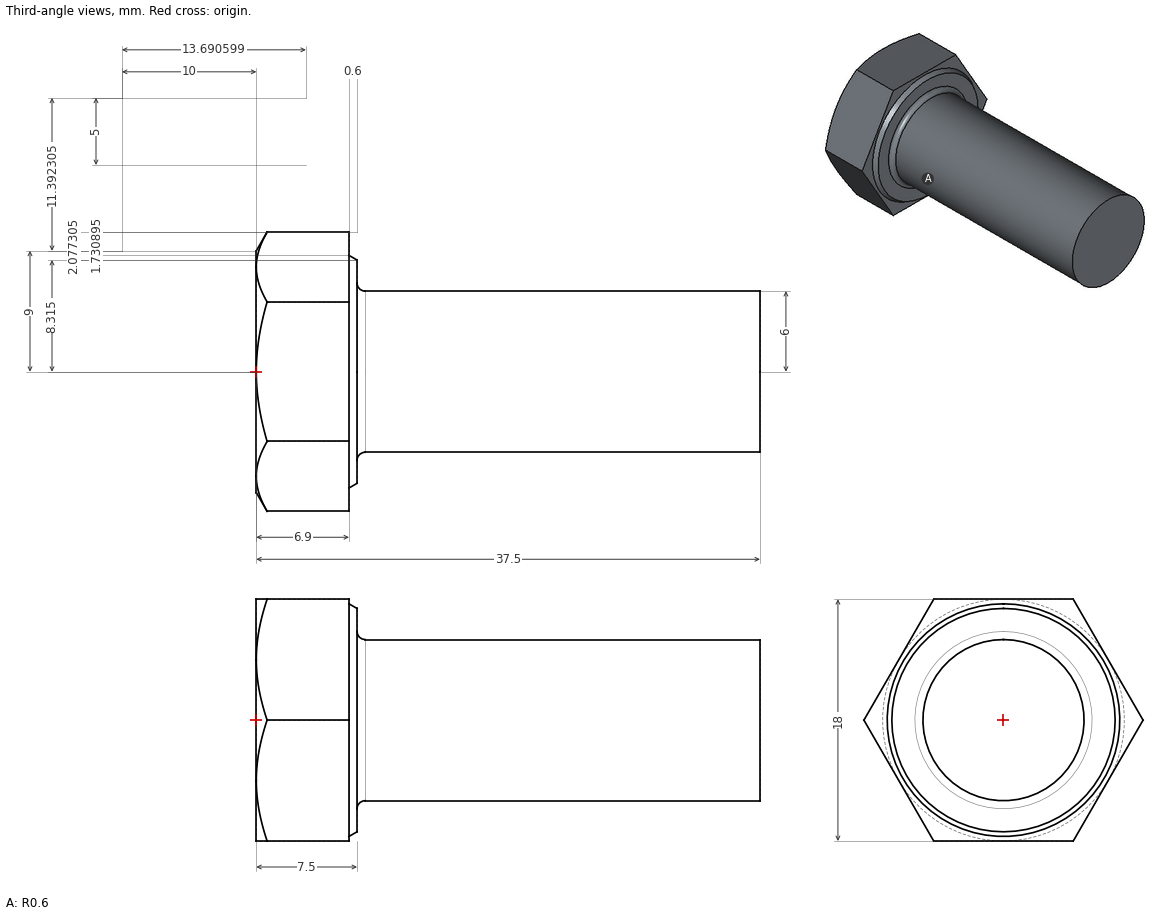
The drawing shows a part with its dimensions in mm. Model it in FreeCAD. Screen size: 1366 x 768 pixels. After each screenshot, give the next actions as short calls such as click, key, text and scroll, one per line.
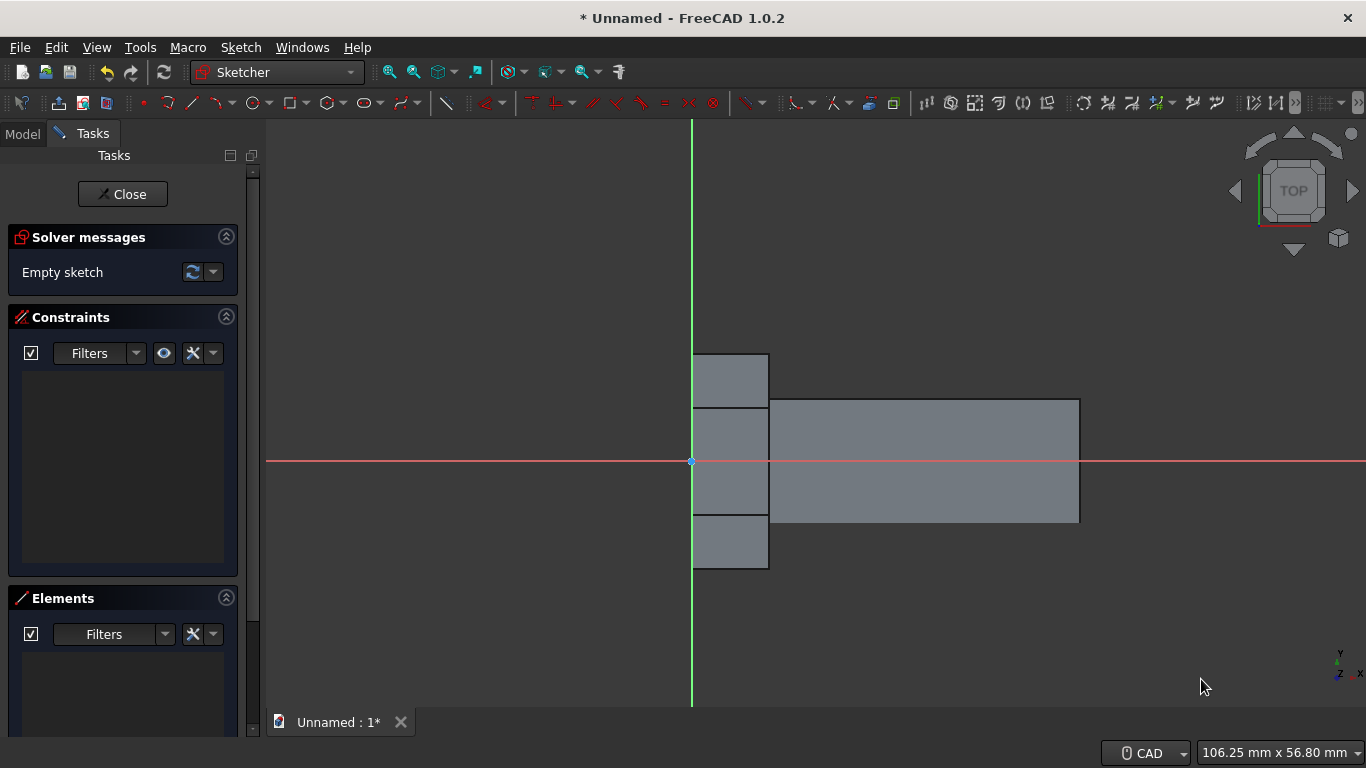
scroll(552, 286, up, 3)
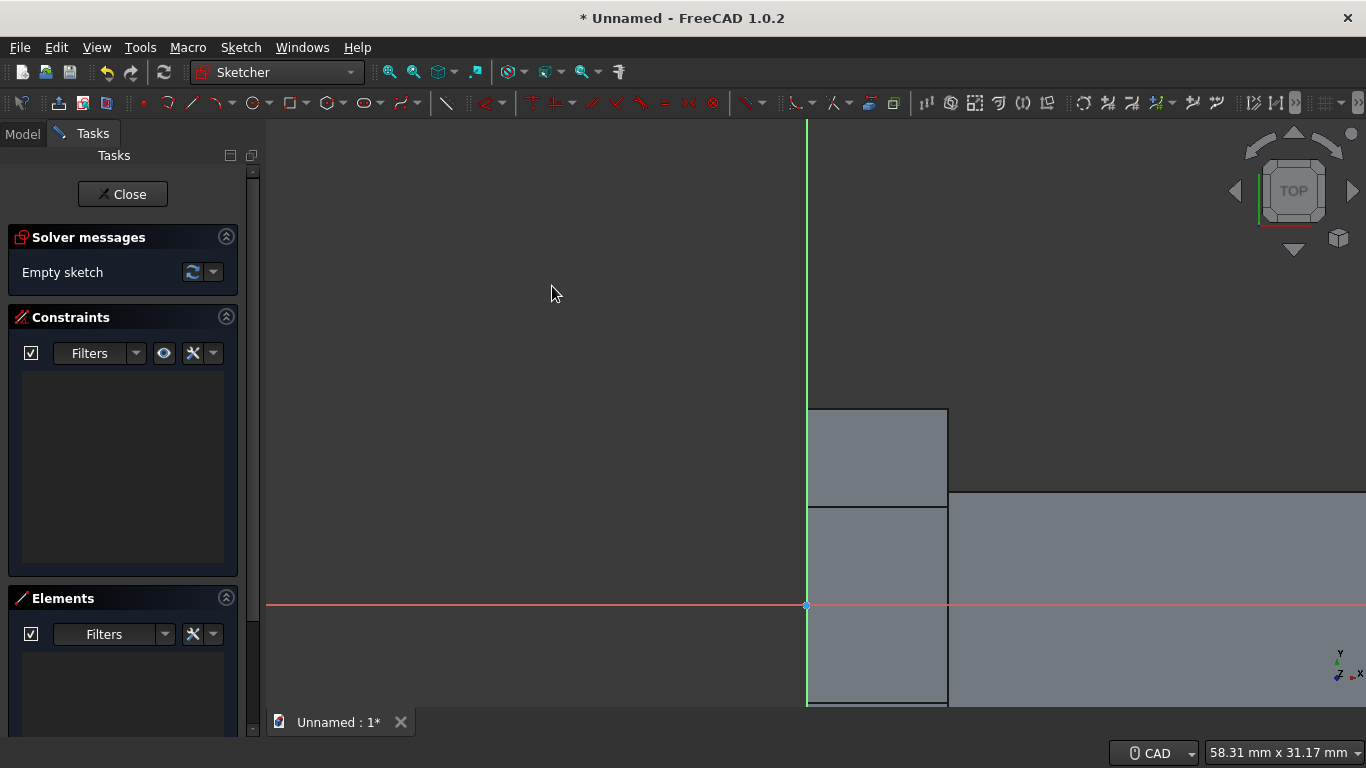
click(168, 104)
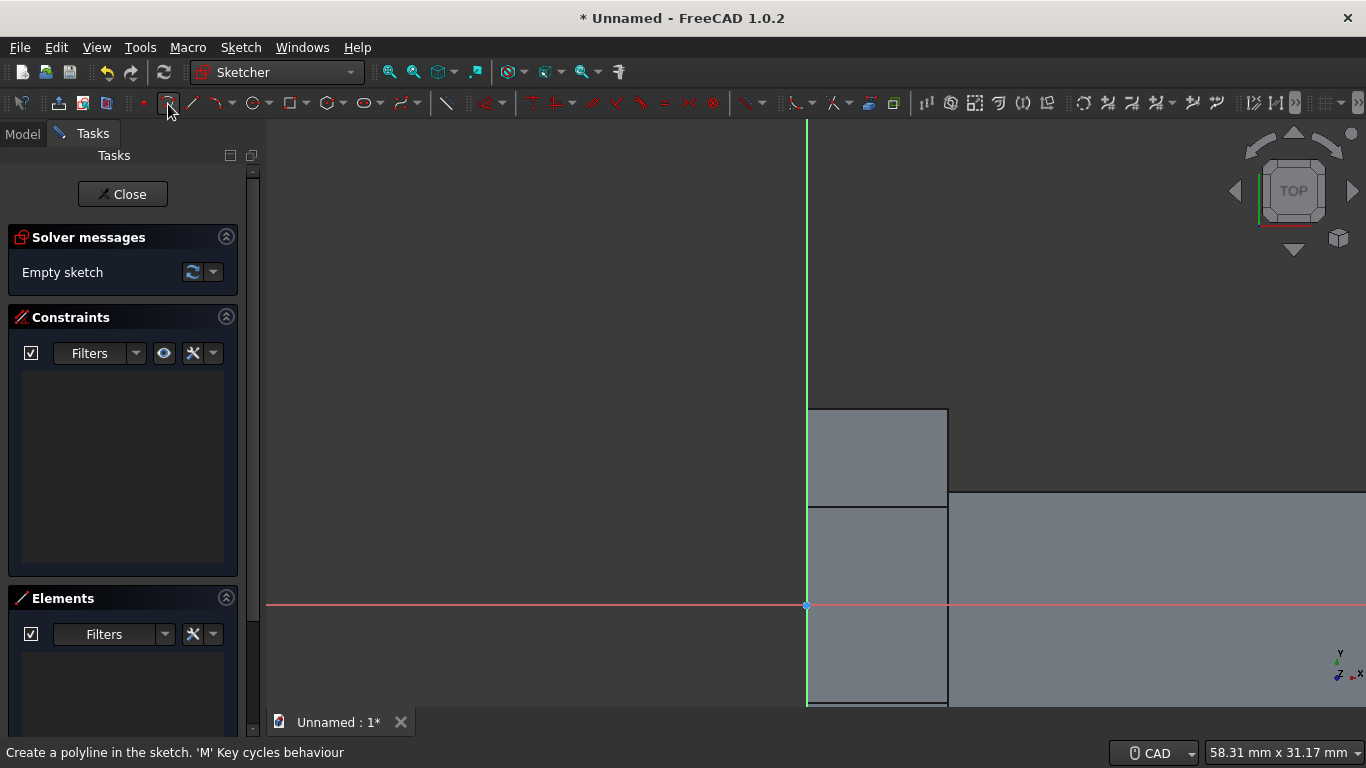
click(807, 436)
click(876, 315)
click(876, 221)
click(618, 221)
click(618, 436)
click(807, 437)
key(Escape)
key(Escape)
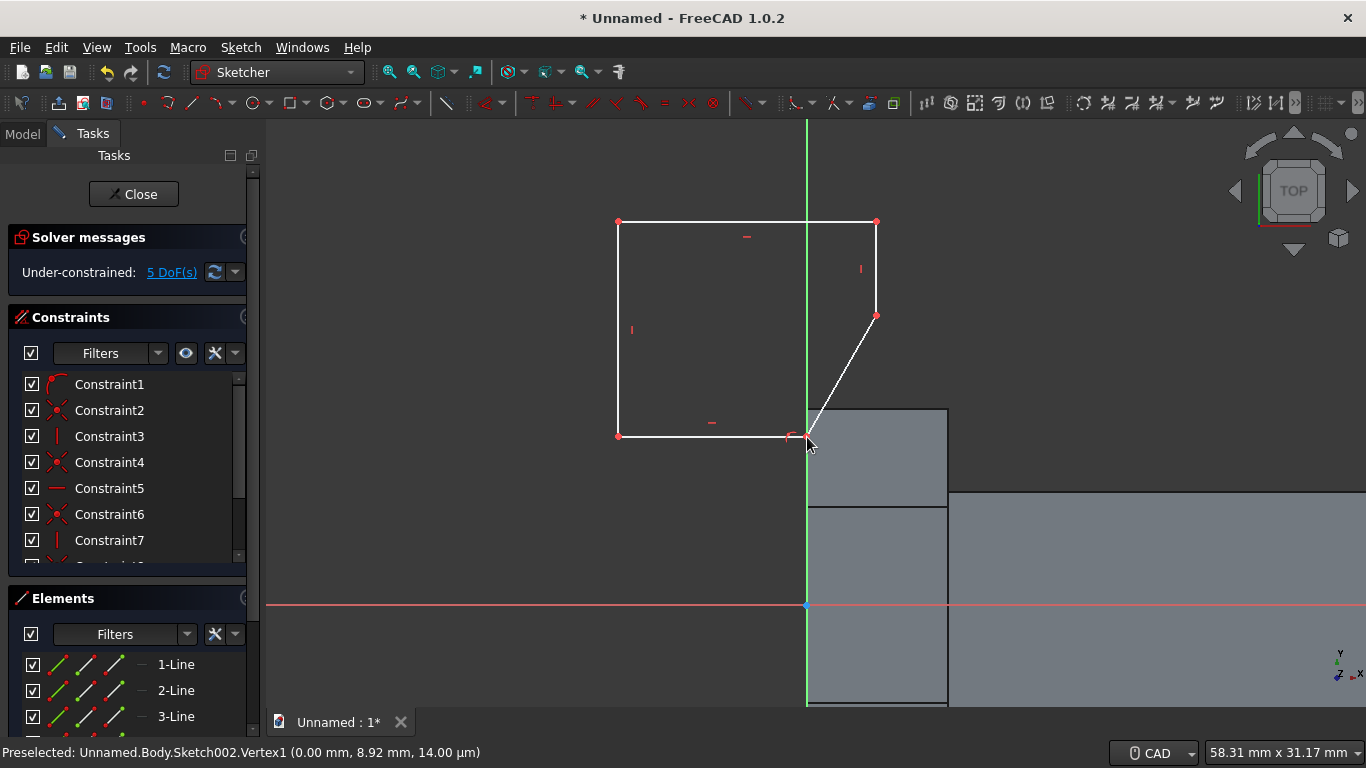
click(876, 288)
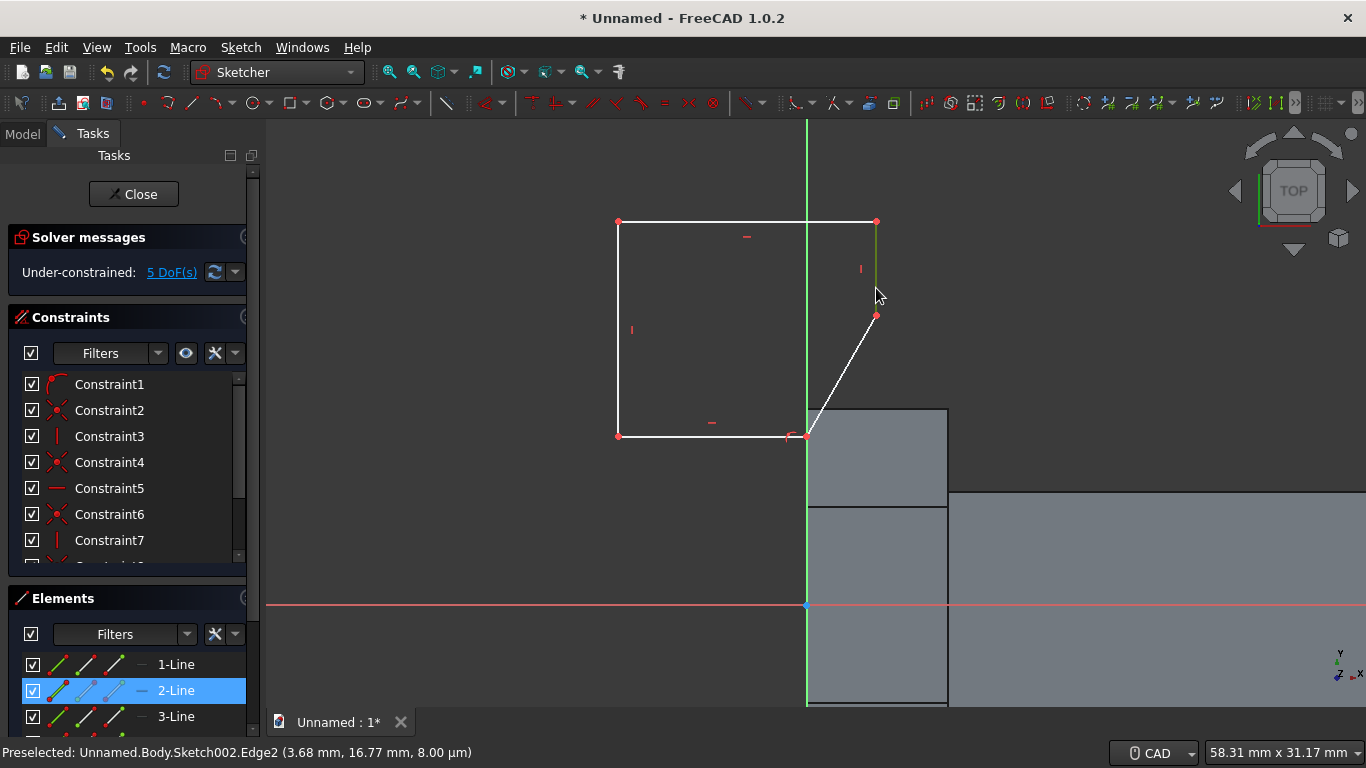
key(i)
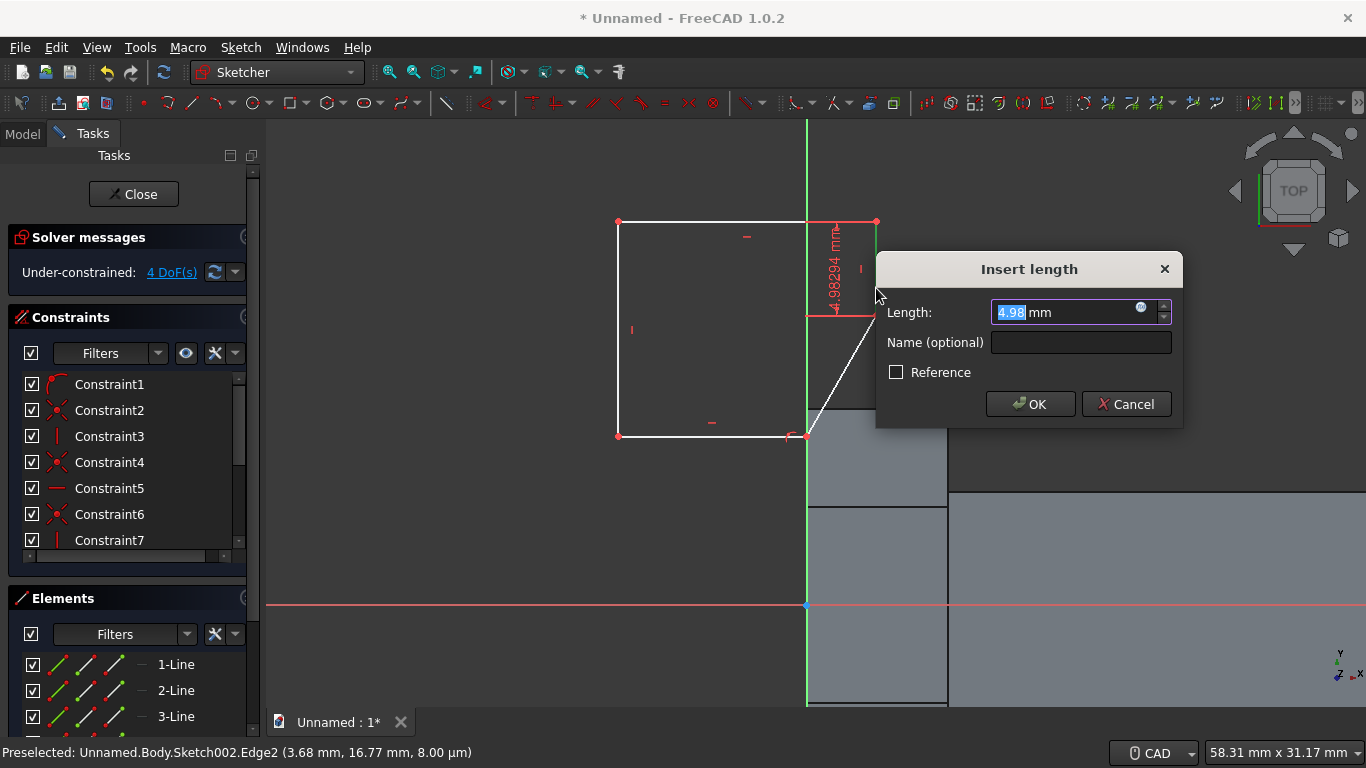
text(5)
key(Return)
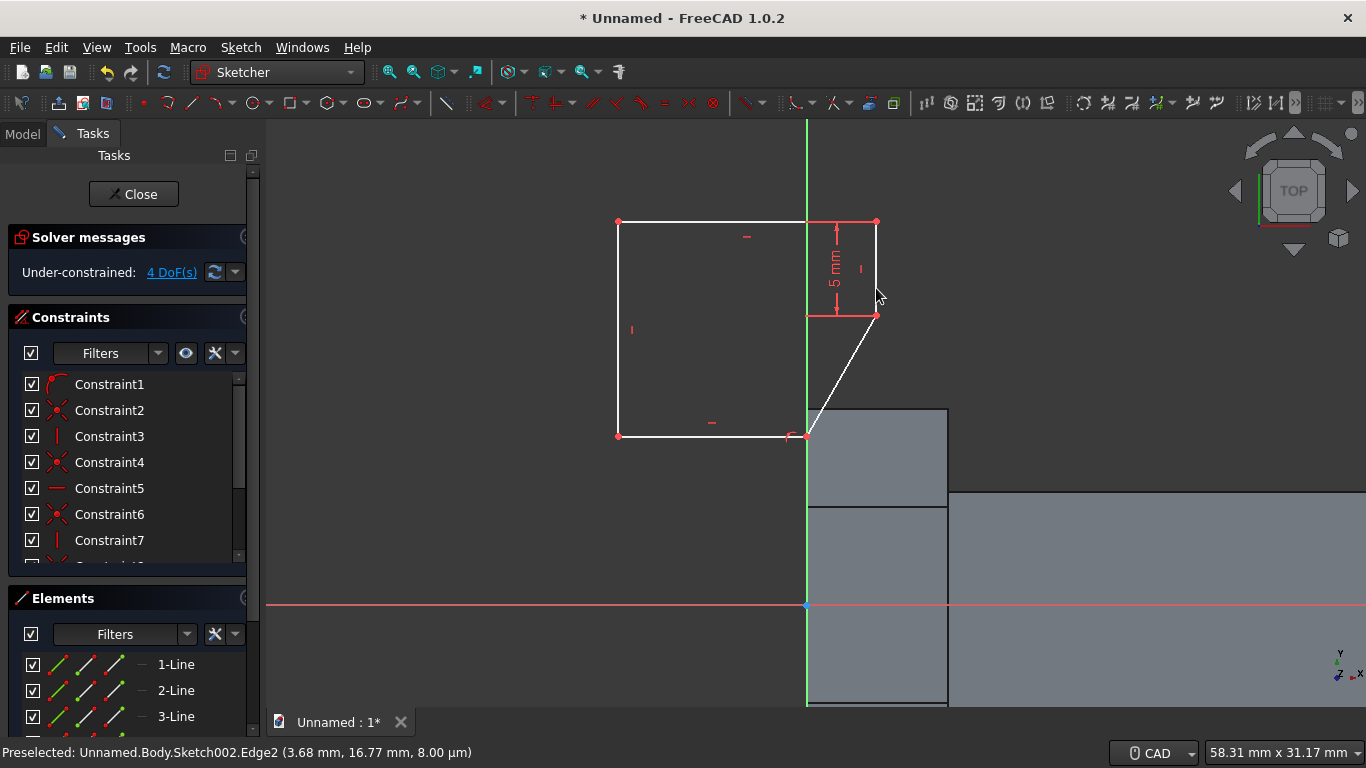
click(675, 437)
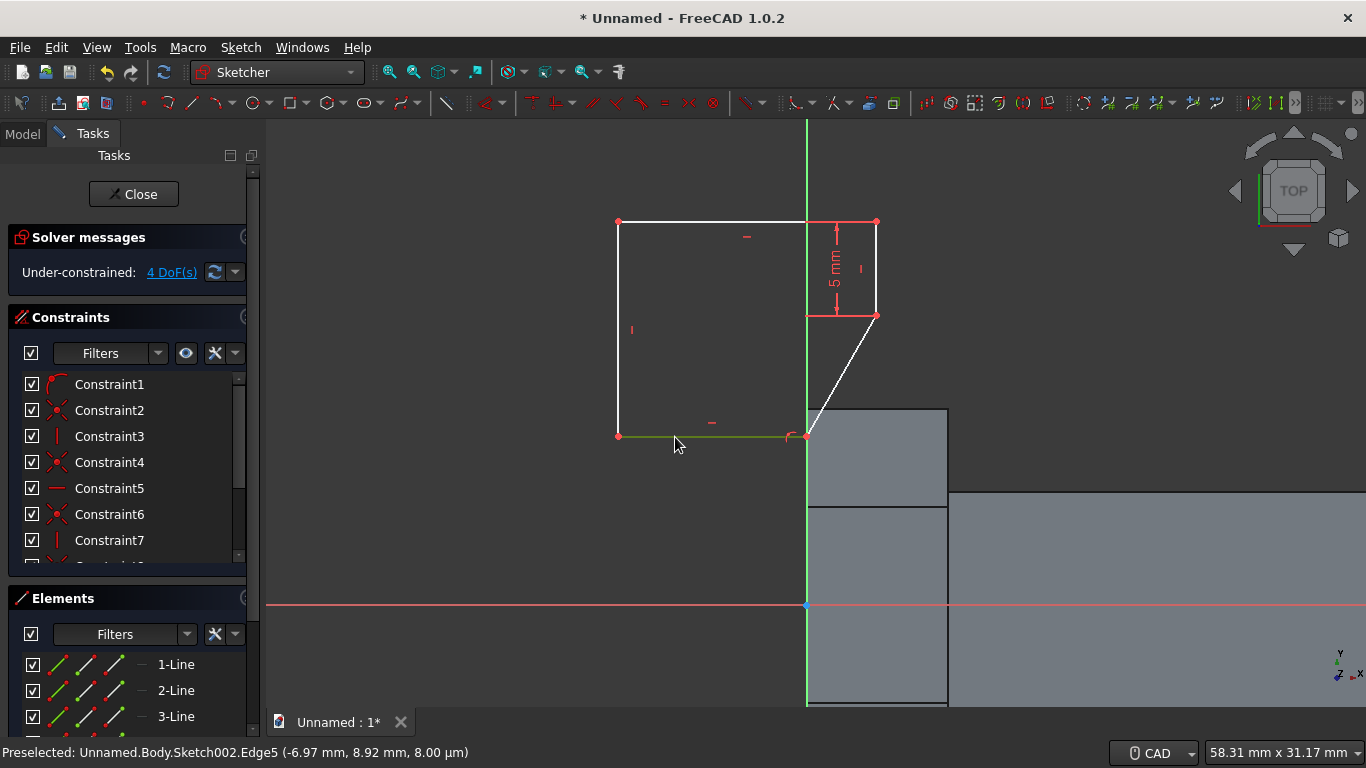
click(504, 104)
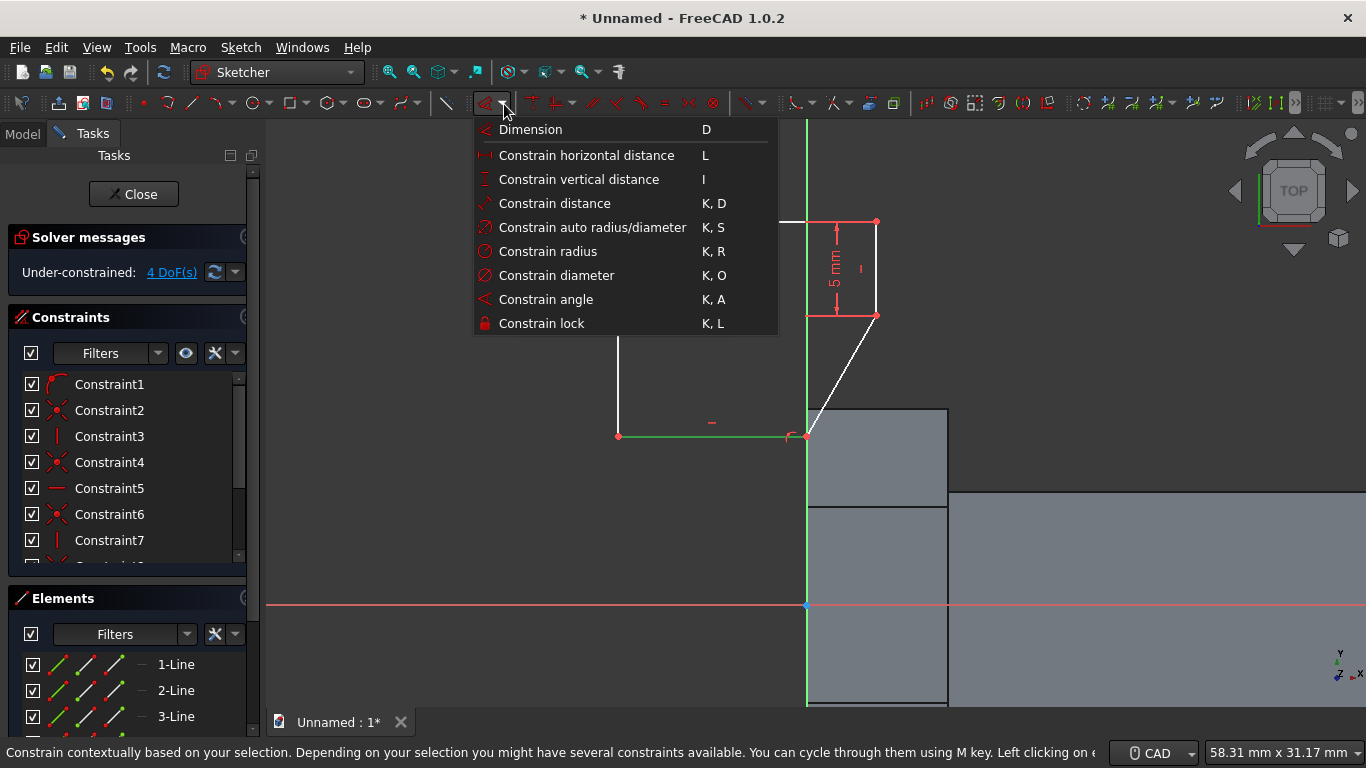
click(626, 155)